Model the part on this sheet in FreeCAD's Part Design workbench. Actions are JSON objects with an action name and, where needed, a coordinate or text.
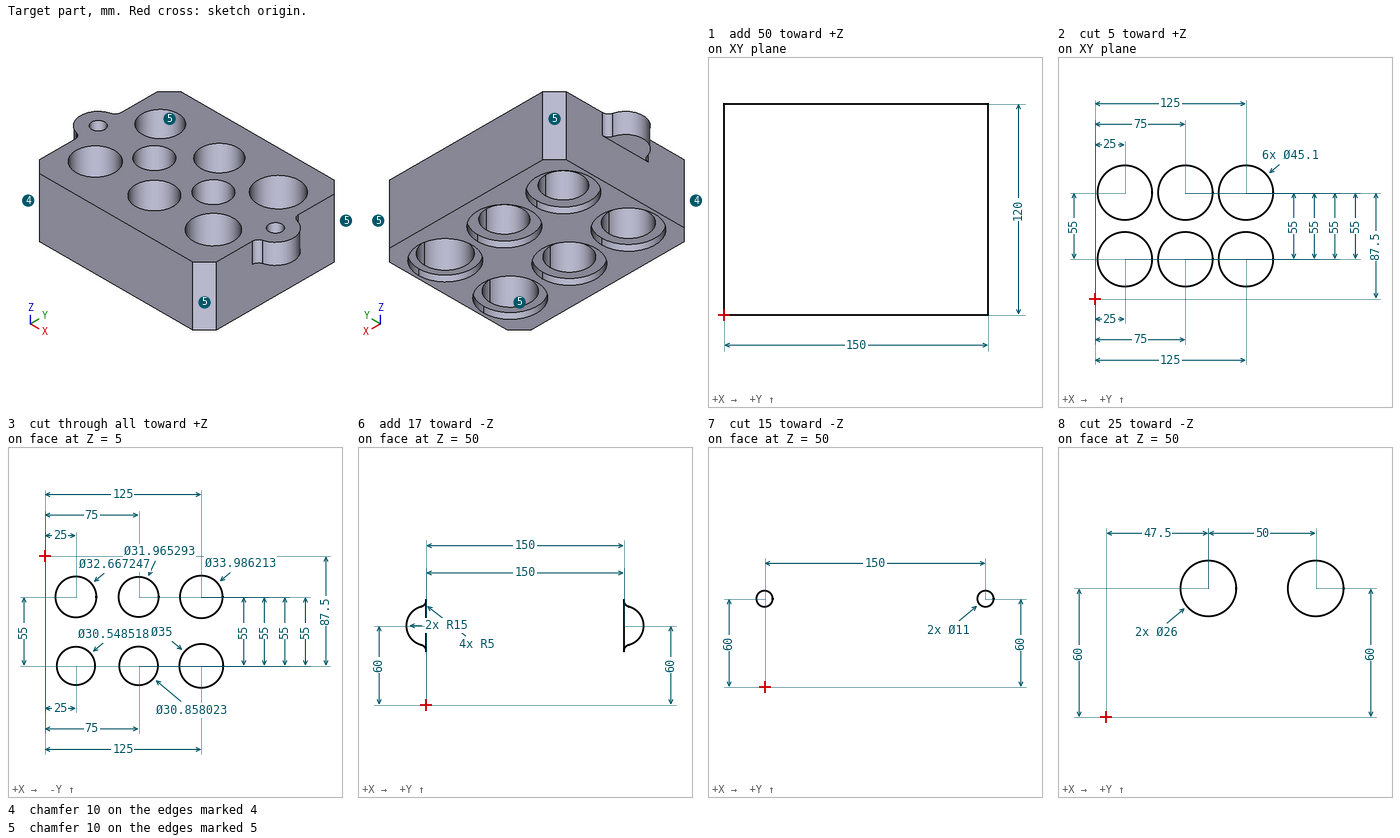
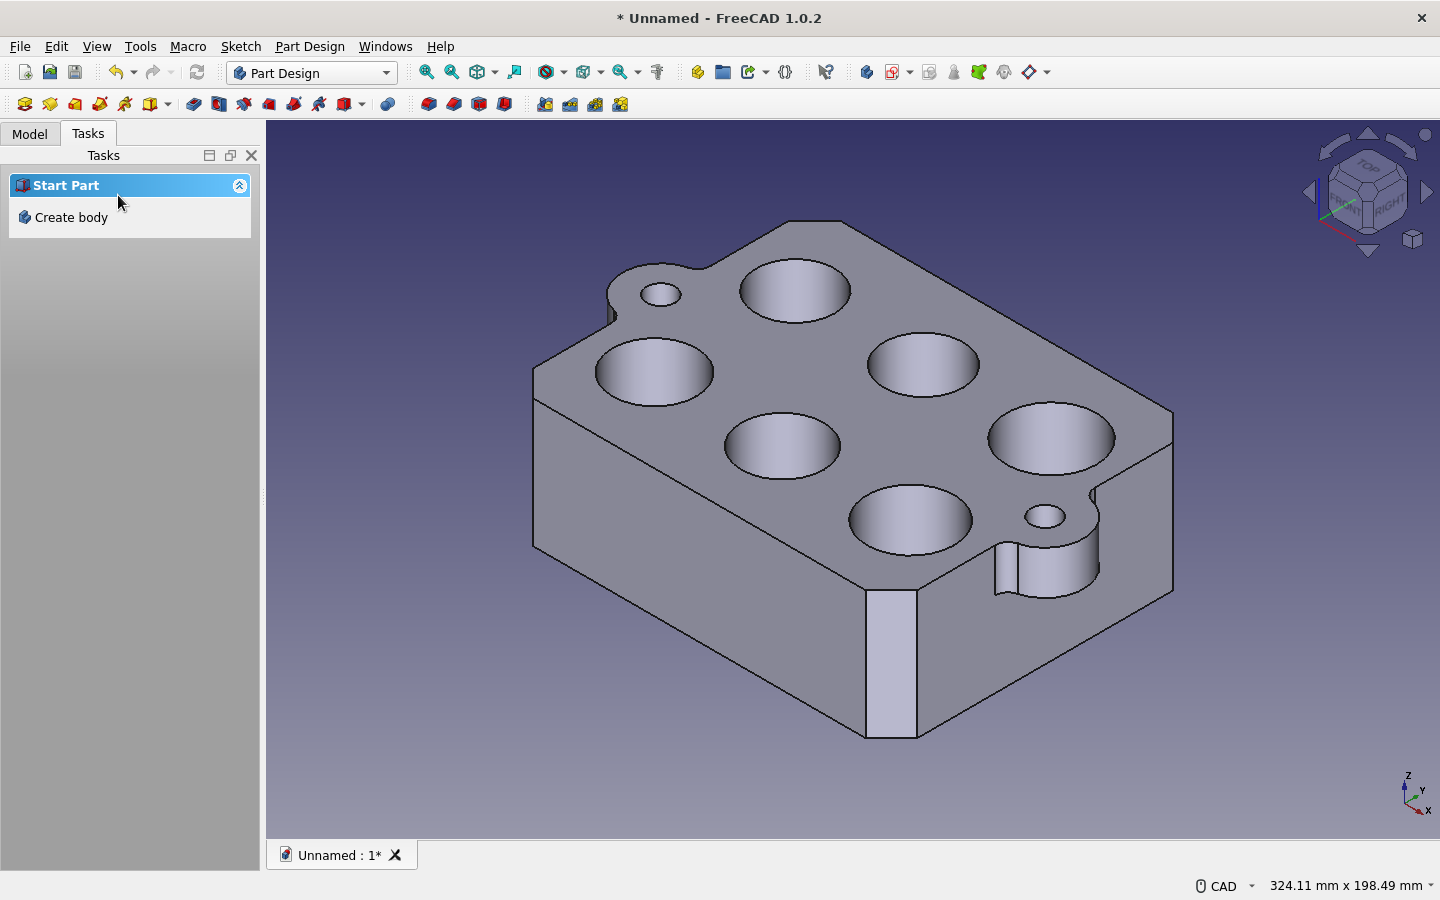
{"action": "left_click", "coordinate": [787, 367]}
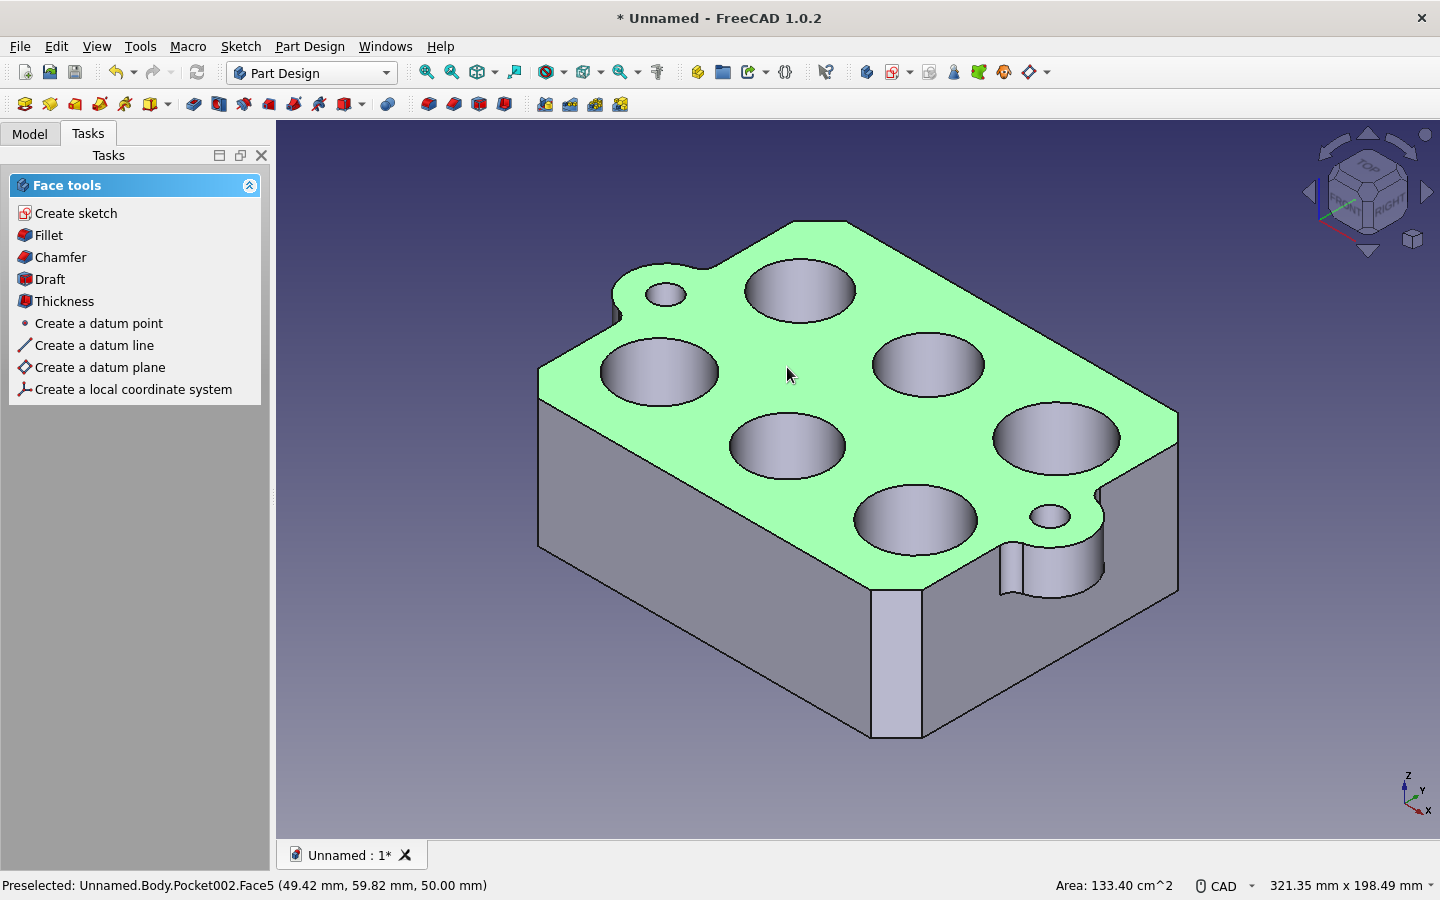
{"action": "left_click", "coordinate": [892, 72]}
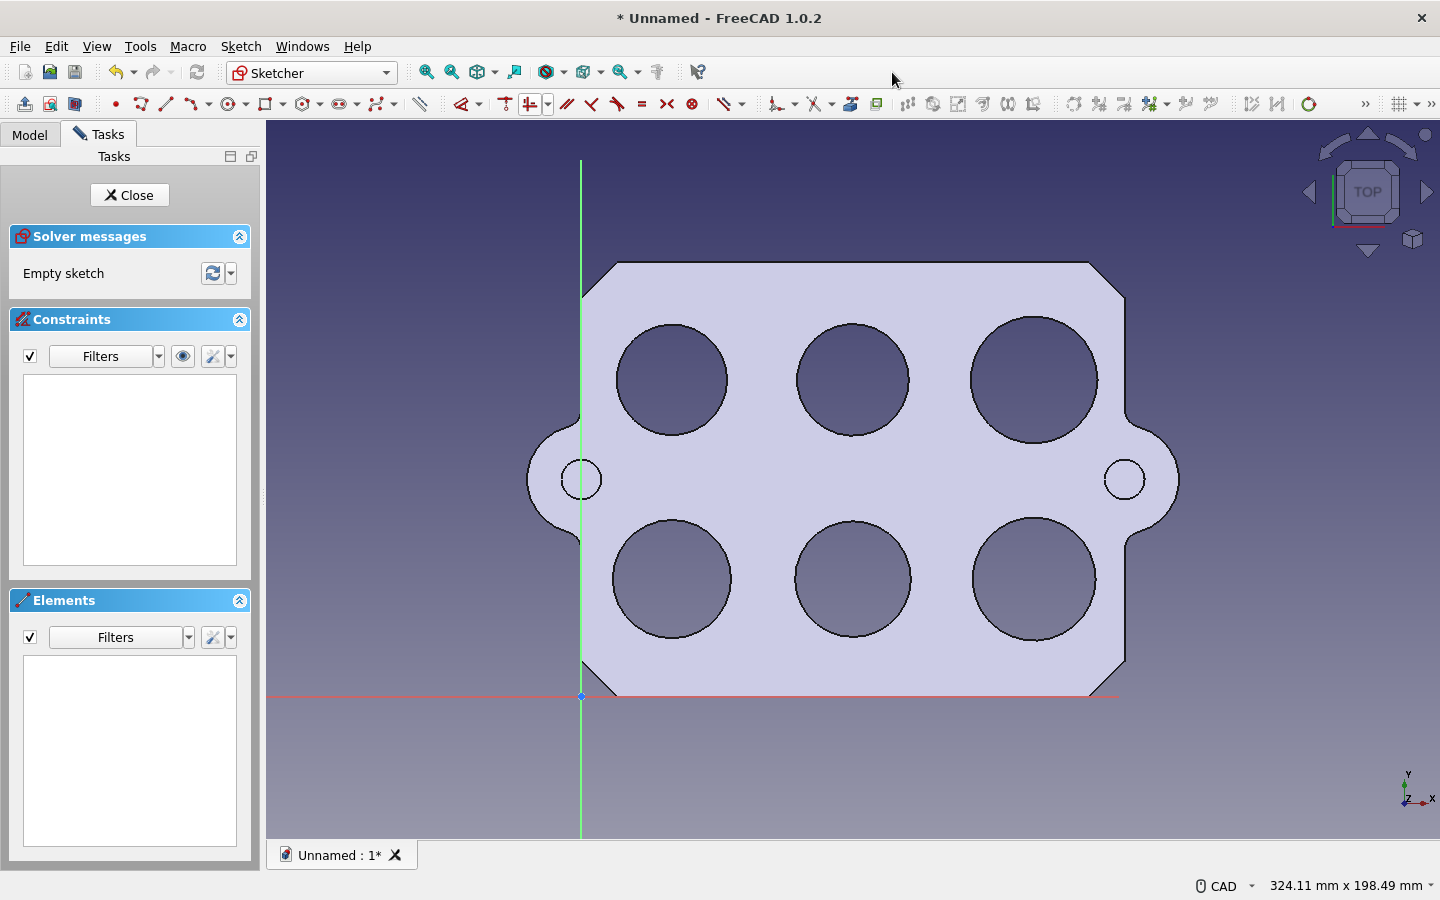
{"action": "scroll", "coordinate": [778, 668], "scroll_direction": "up", "scroll_amount": 3}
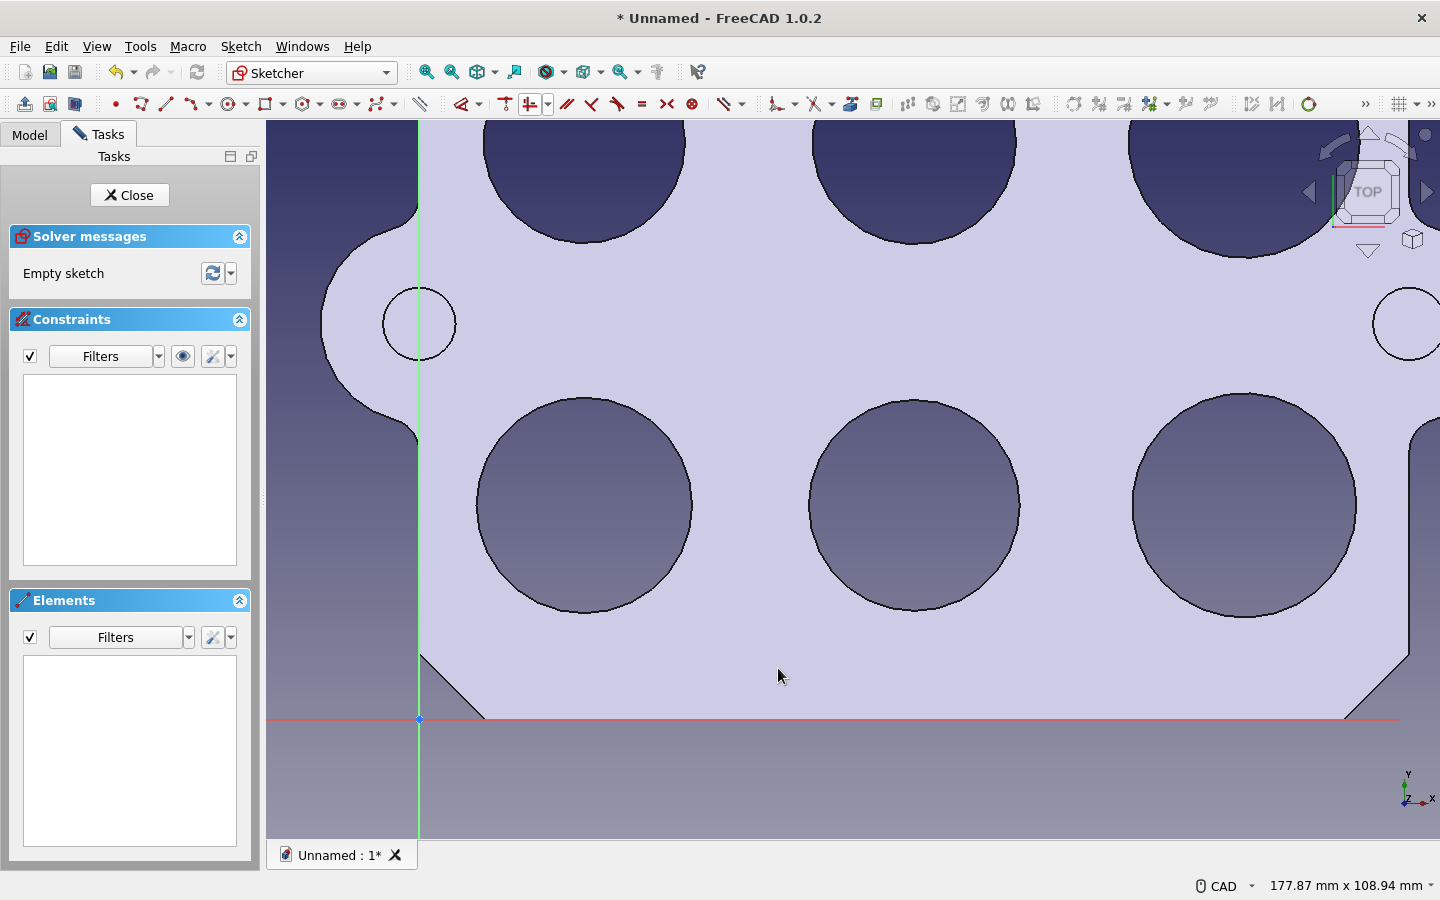
{"action": "left_click", "coordinate": [228, 104]}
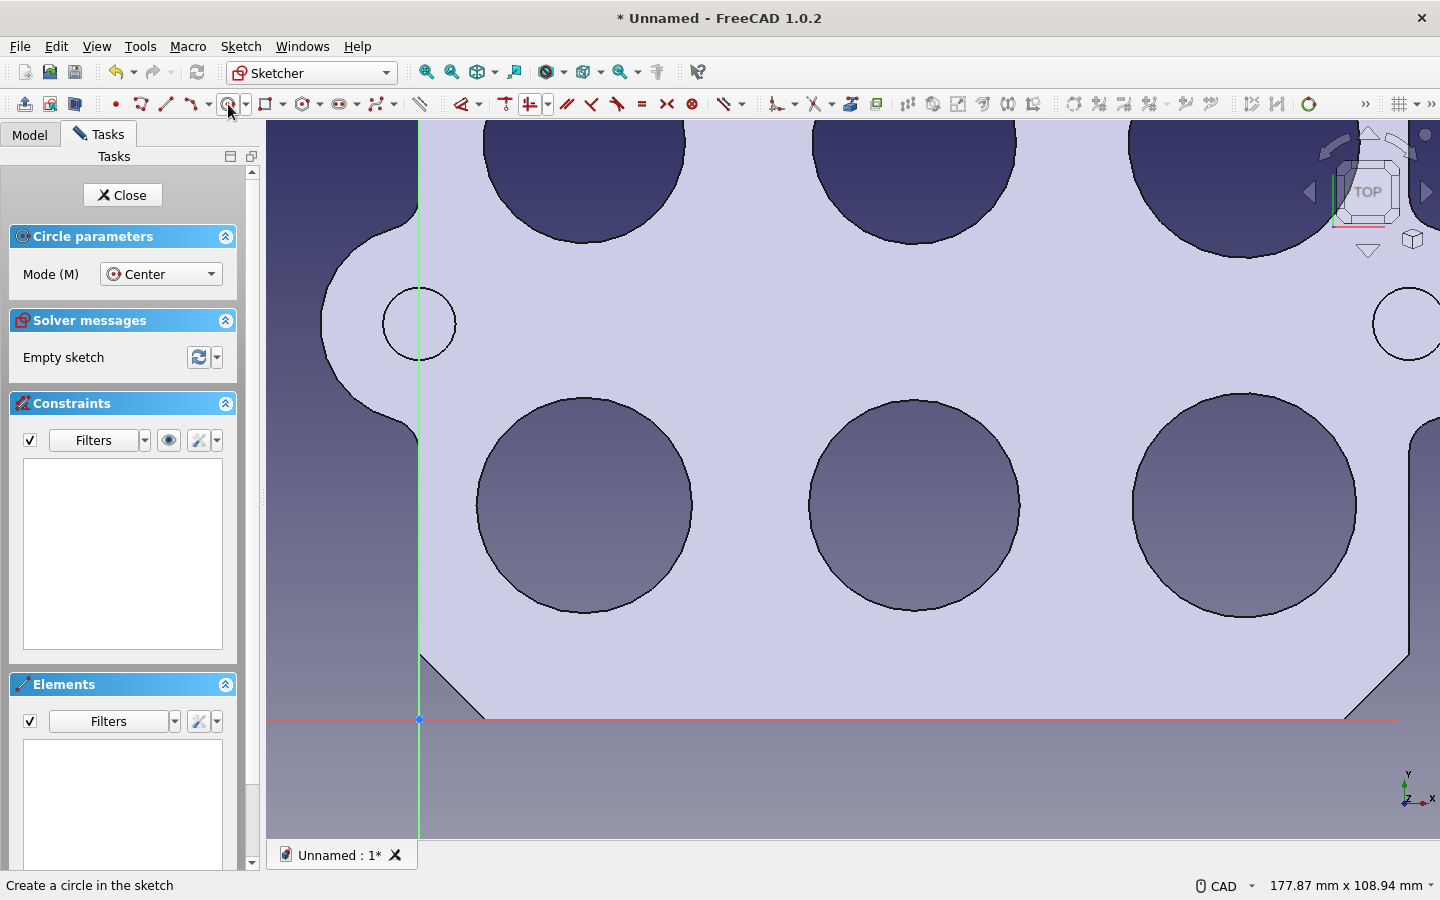
{"action": "left_click", "coordinate": [733, 324]}
{"action": "left_click", "coordinate": [793, 263]}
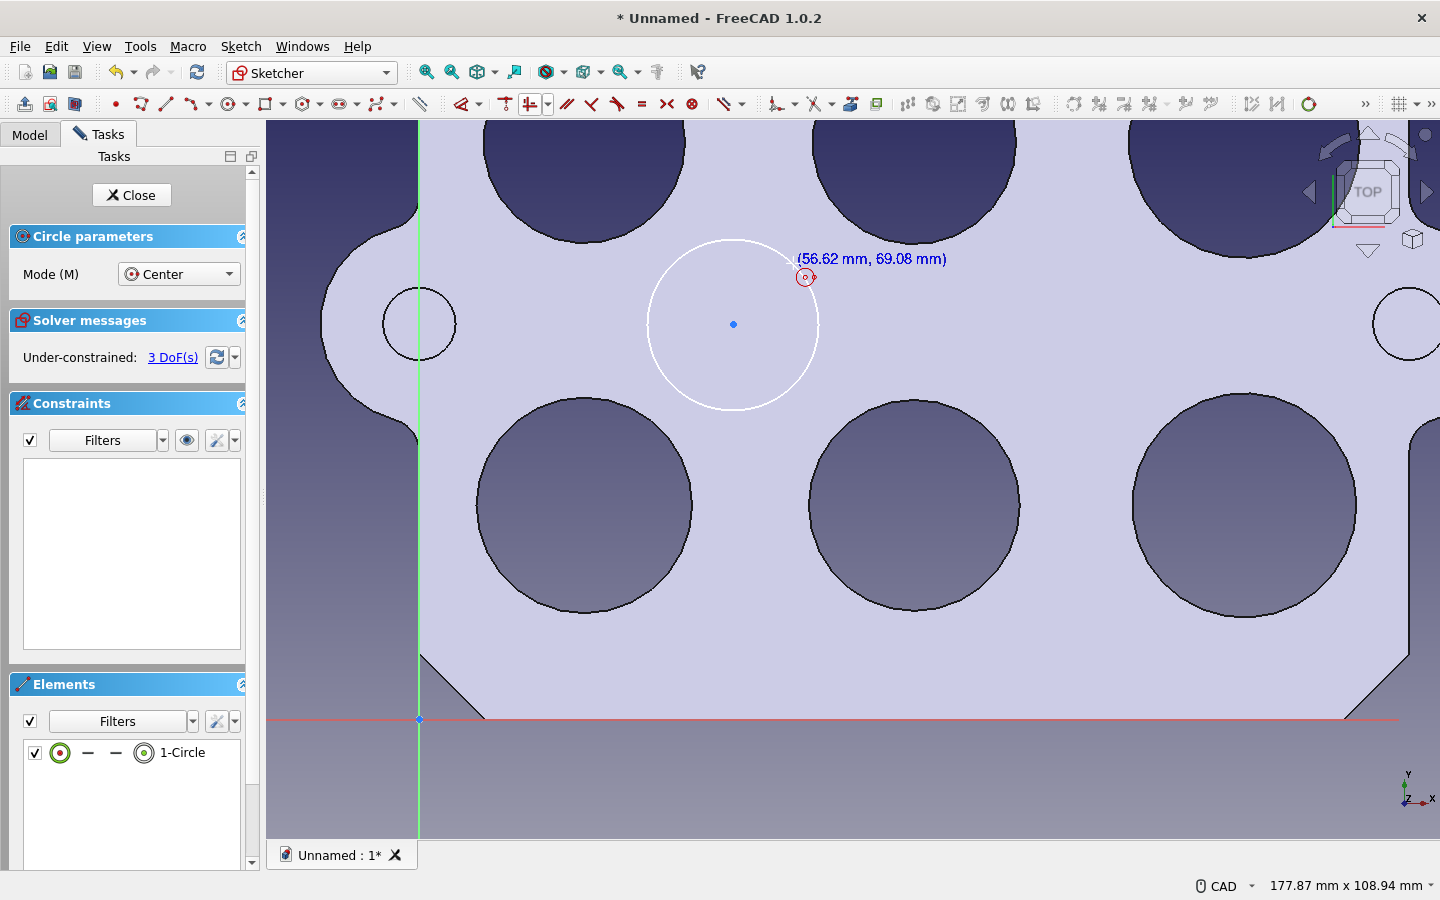
{"action": "left_click", "coordinate": [1063, 324]}
{"action": "left_click", "coordinate": [1123, 263]}
{"action": "key", "text": "Escape"}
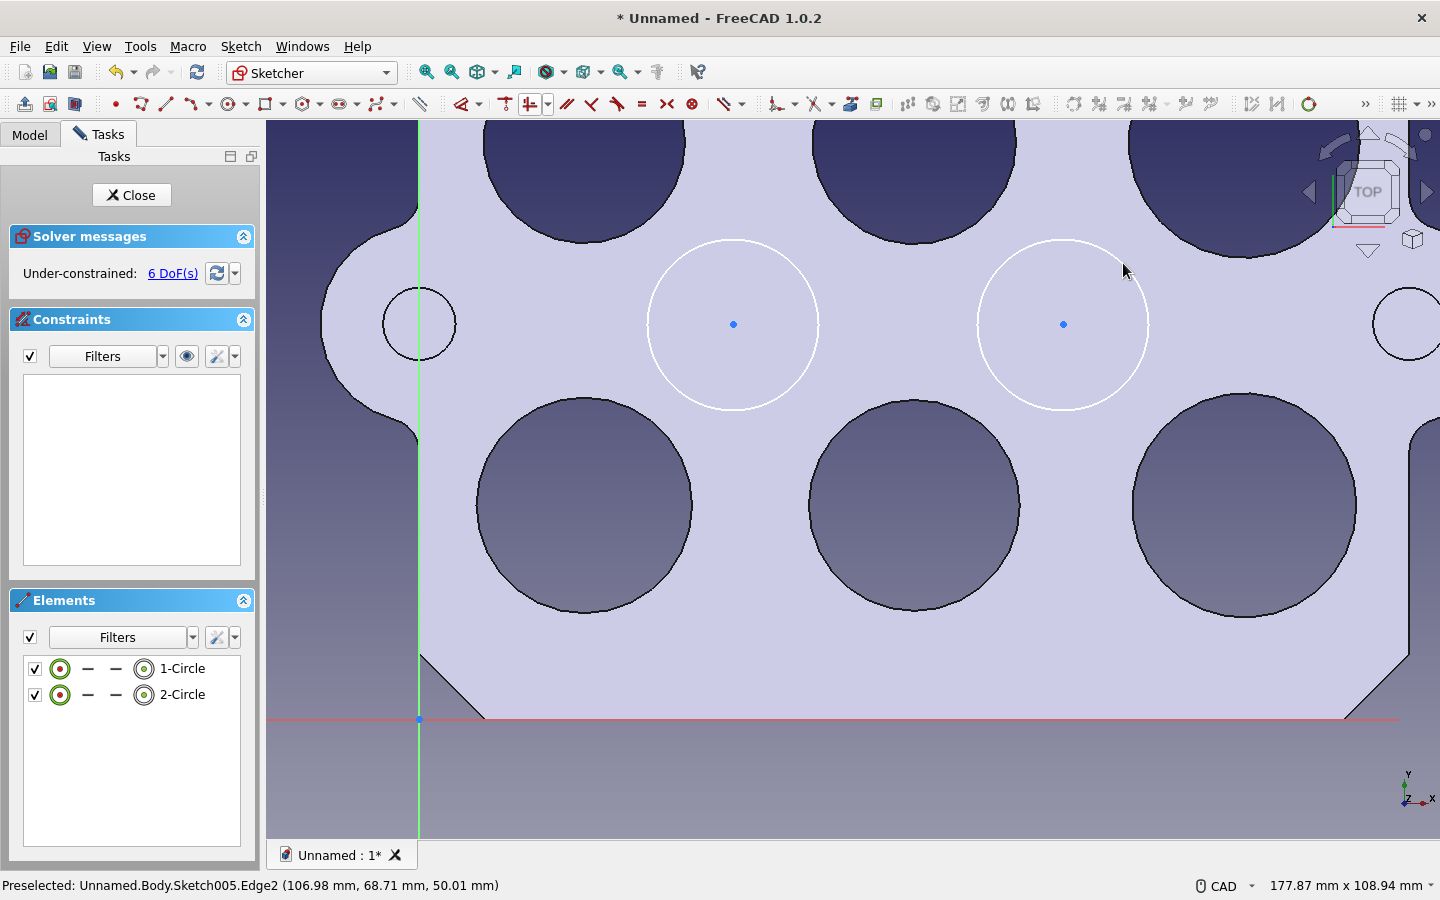
{"action": "left_click", "coordinate": [793, 264]}